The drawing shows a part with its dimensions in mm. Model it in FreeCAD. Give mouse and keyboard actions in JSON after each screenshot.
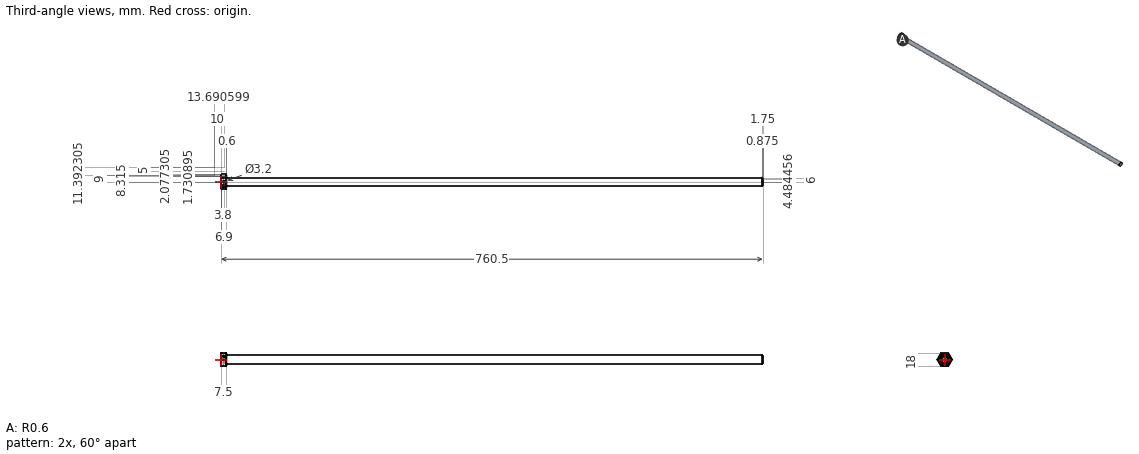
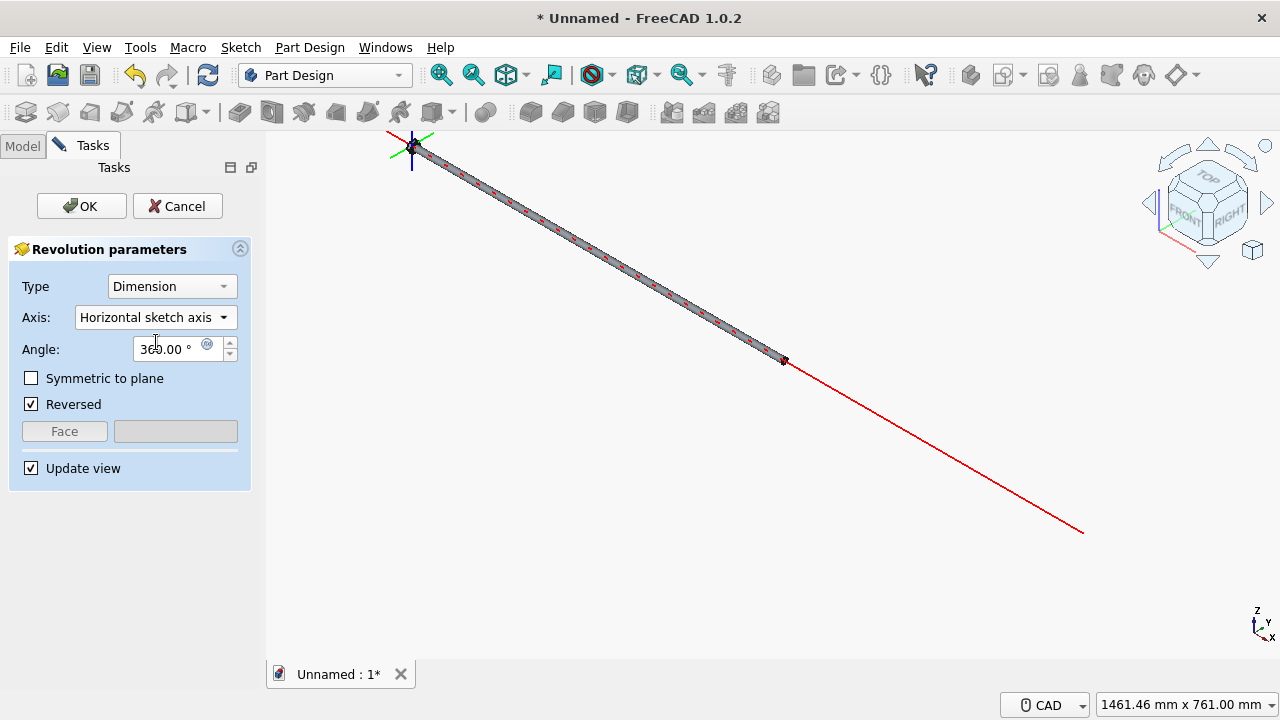
{"action": "left_click", "coordinate": [82, 206]}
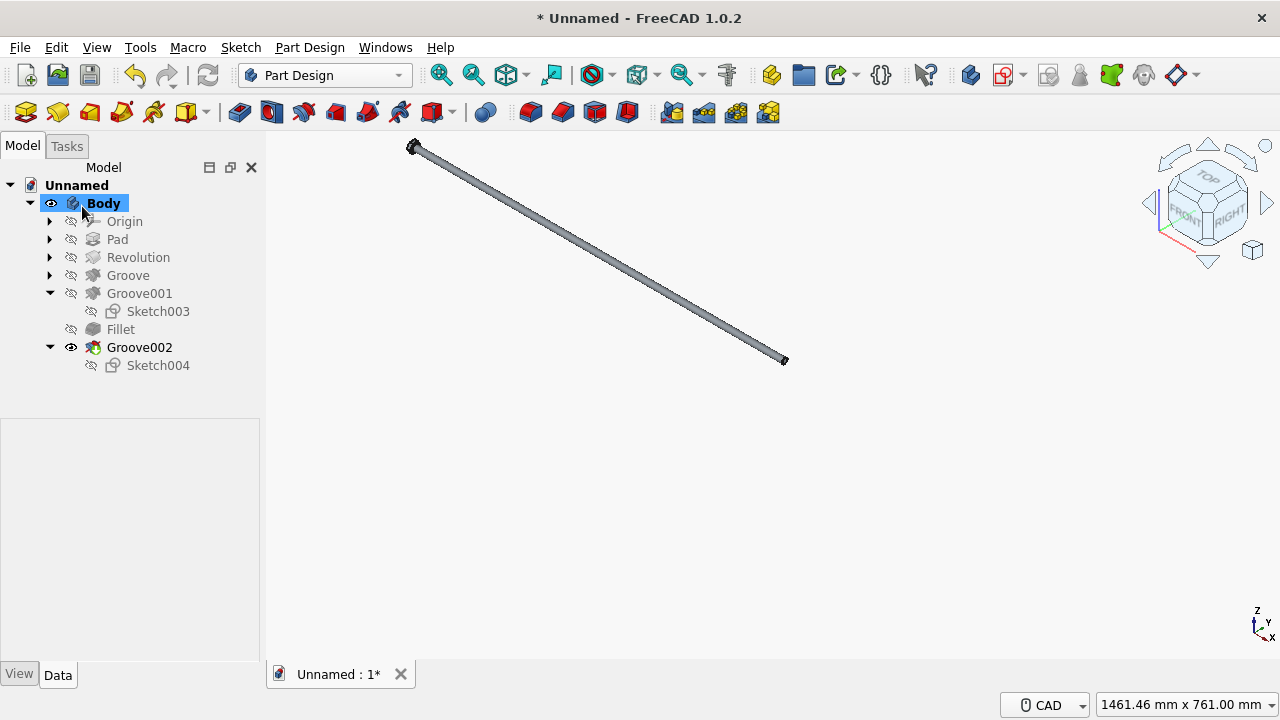
{"action": "key", "text": "v f"}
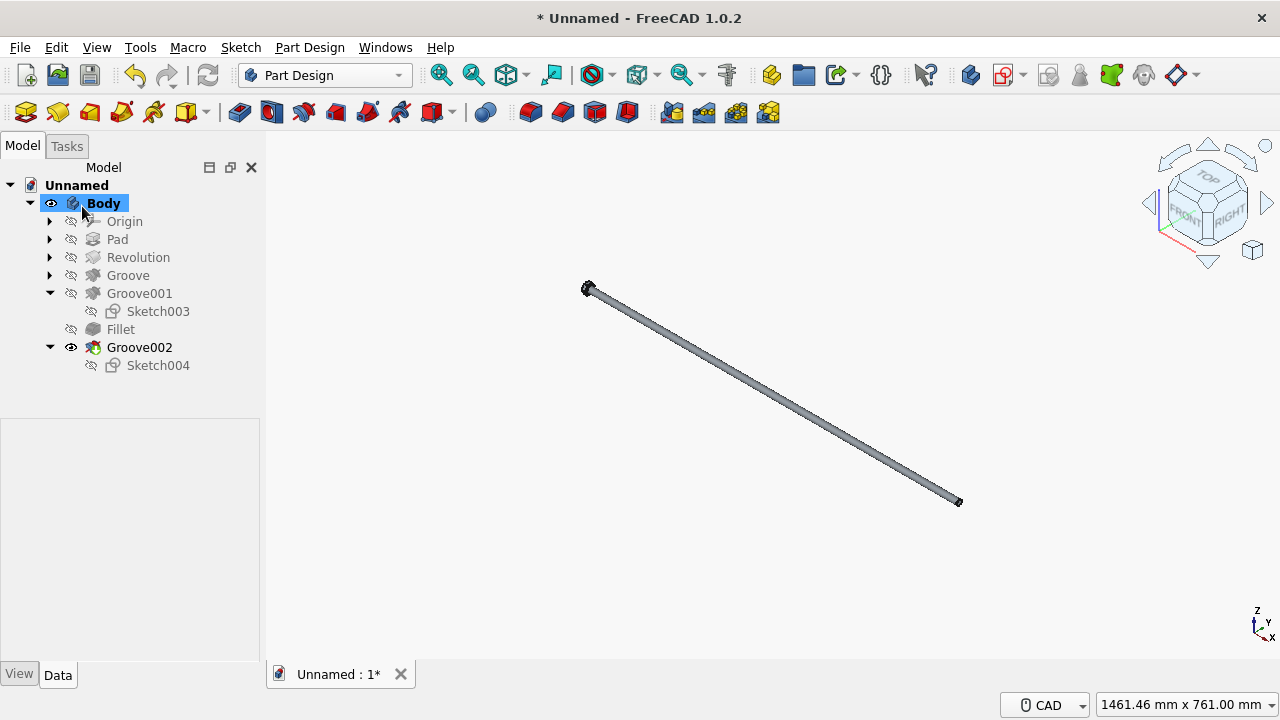
{"action": "left_click", "coordinate": [1004, 76]}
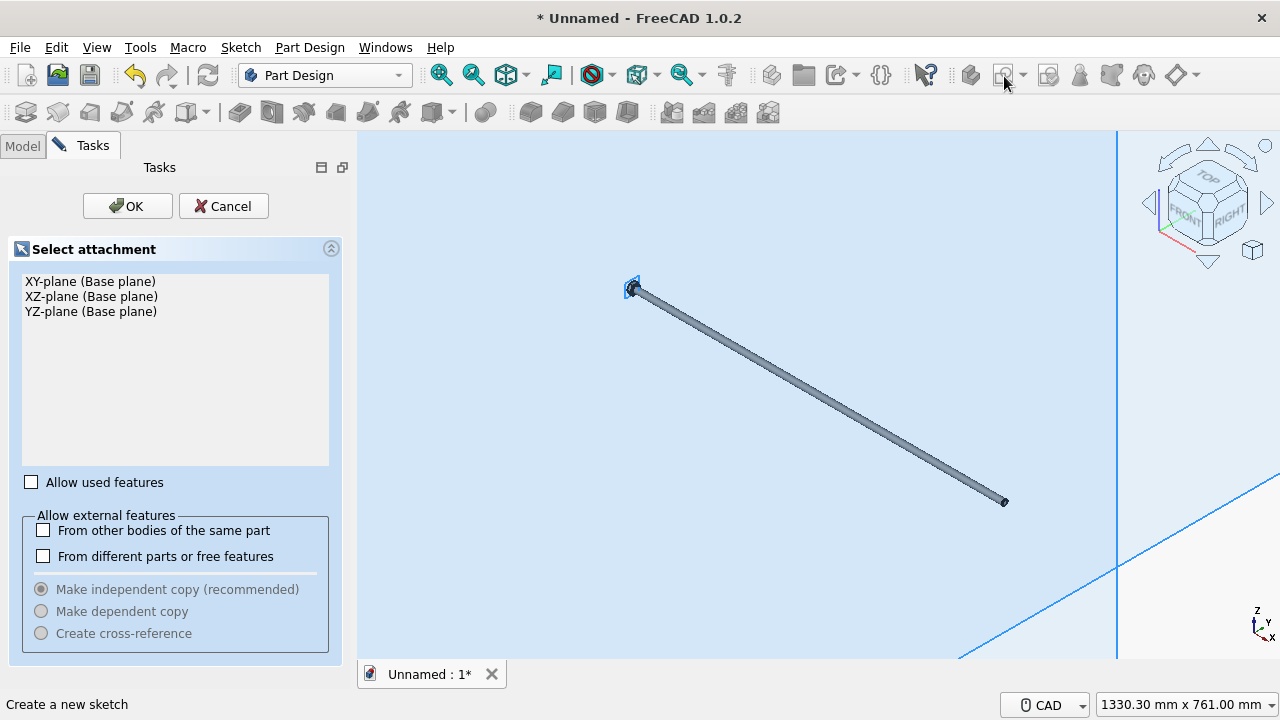
{"action": "left_click", "coordinate": [82, 282]}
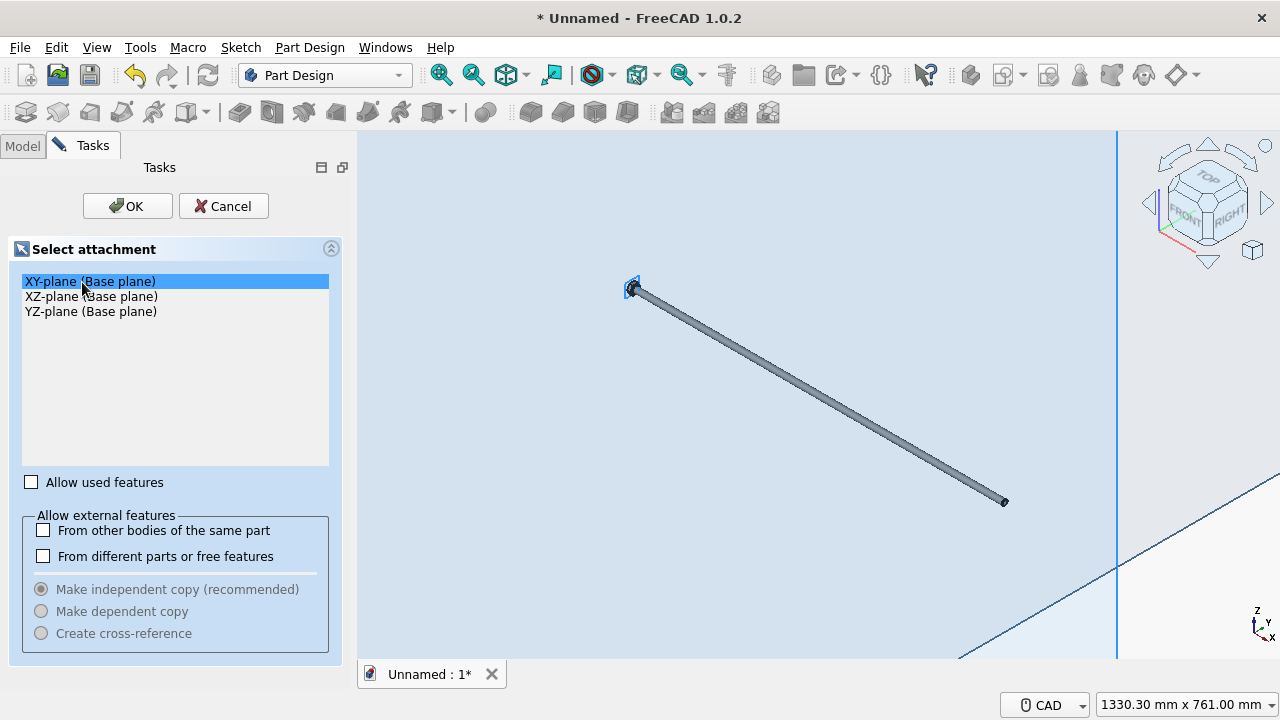
{"action": "left_click", "coordinate": [128, 206]}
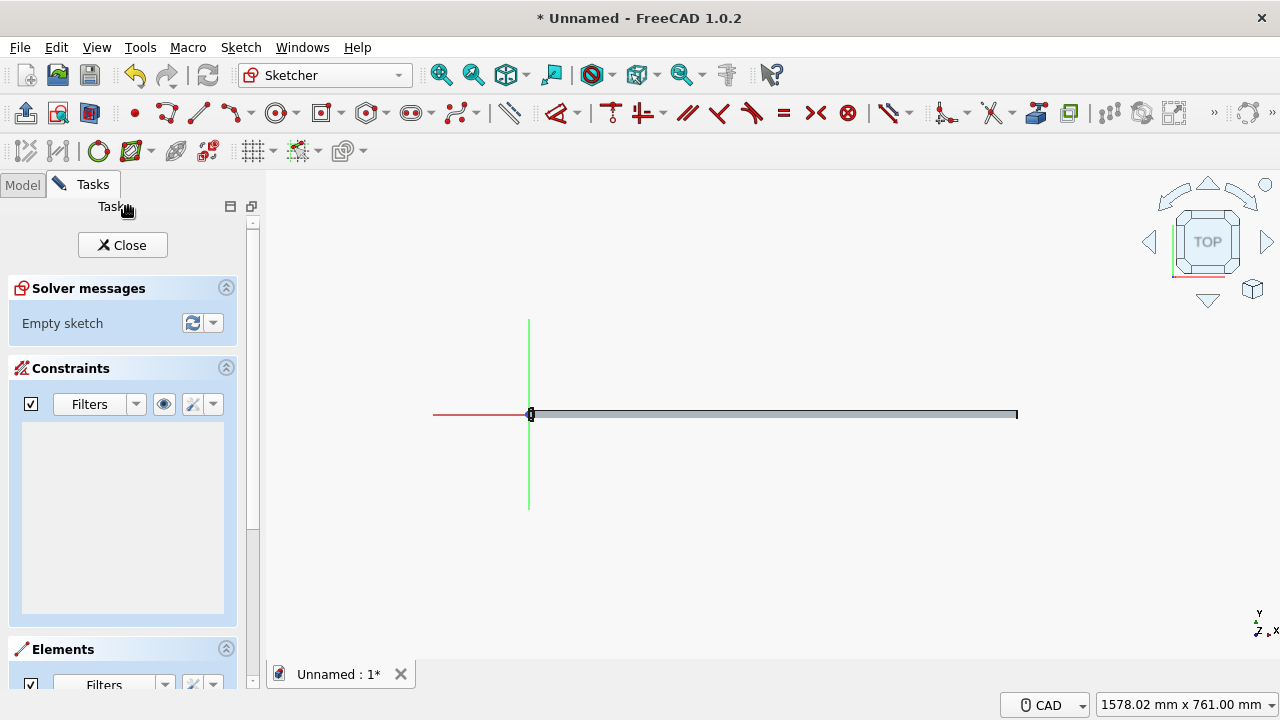
{"action": "key", "text": "q s"}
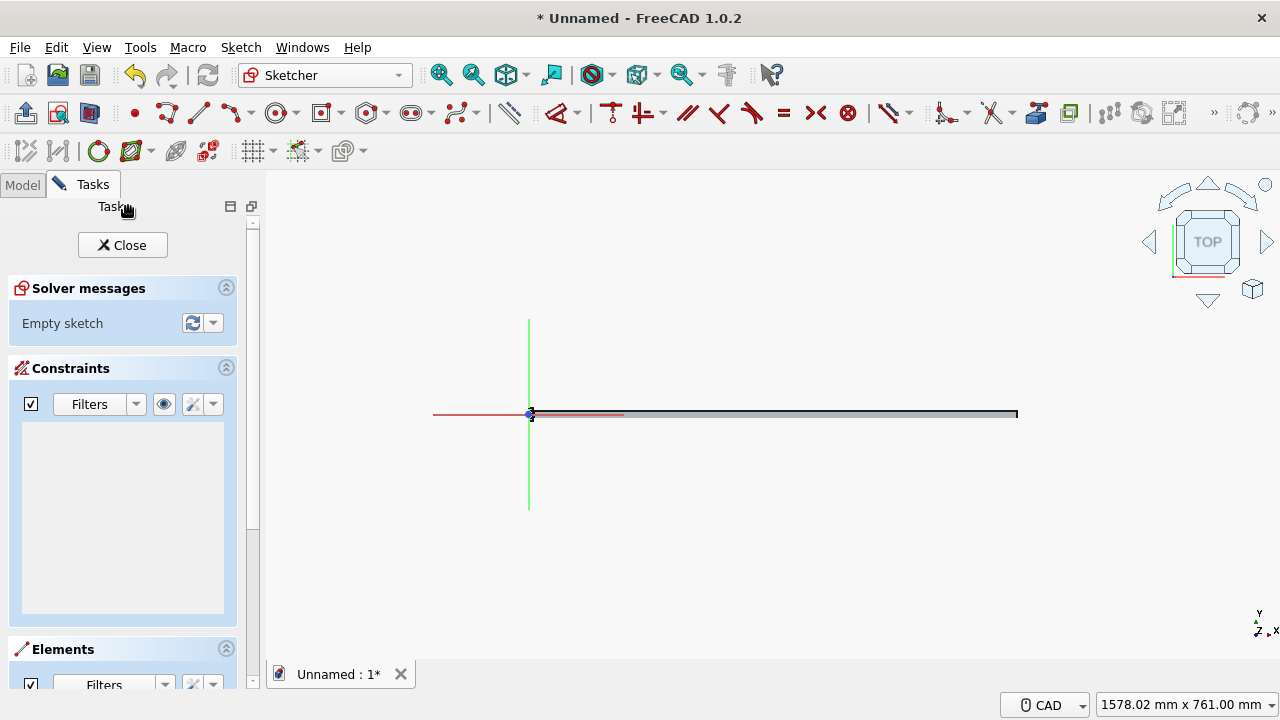
{"action": "scroll", "coordinate": [521, 414], "scroll_direction": "up", "scroll_amount": 15}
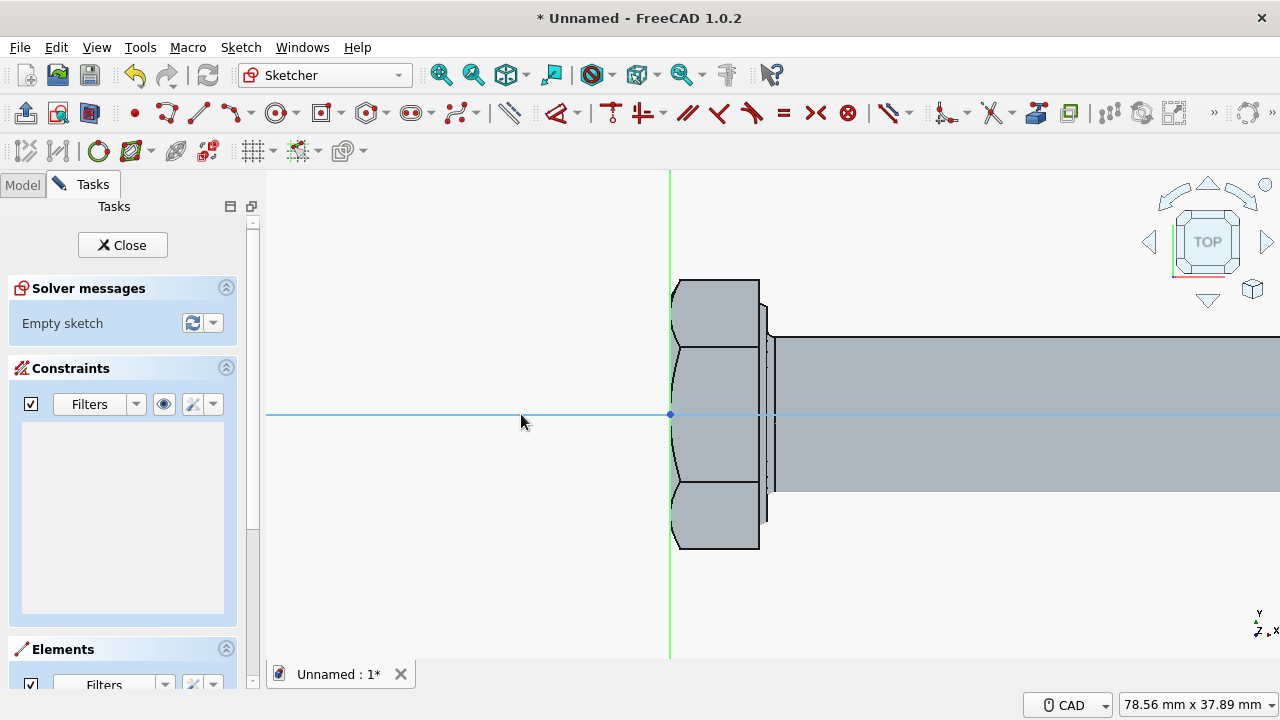
{"action": "scroll", "coordinate": [705, 414], "scroll_direction": "up", "scroll_amount": 10}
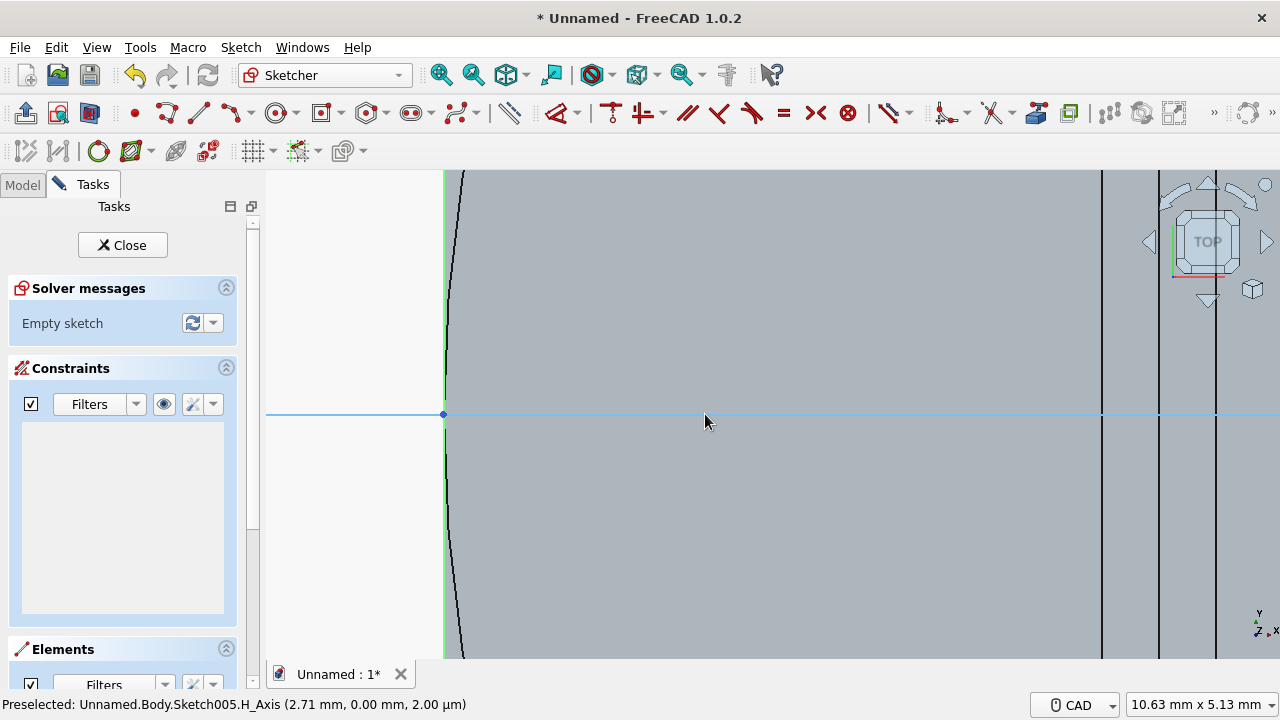
{"action": "key", "text": "g c"}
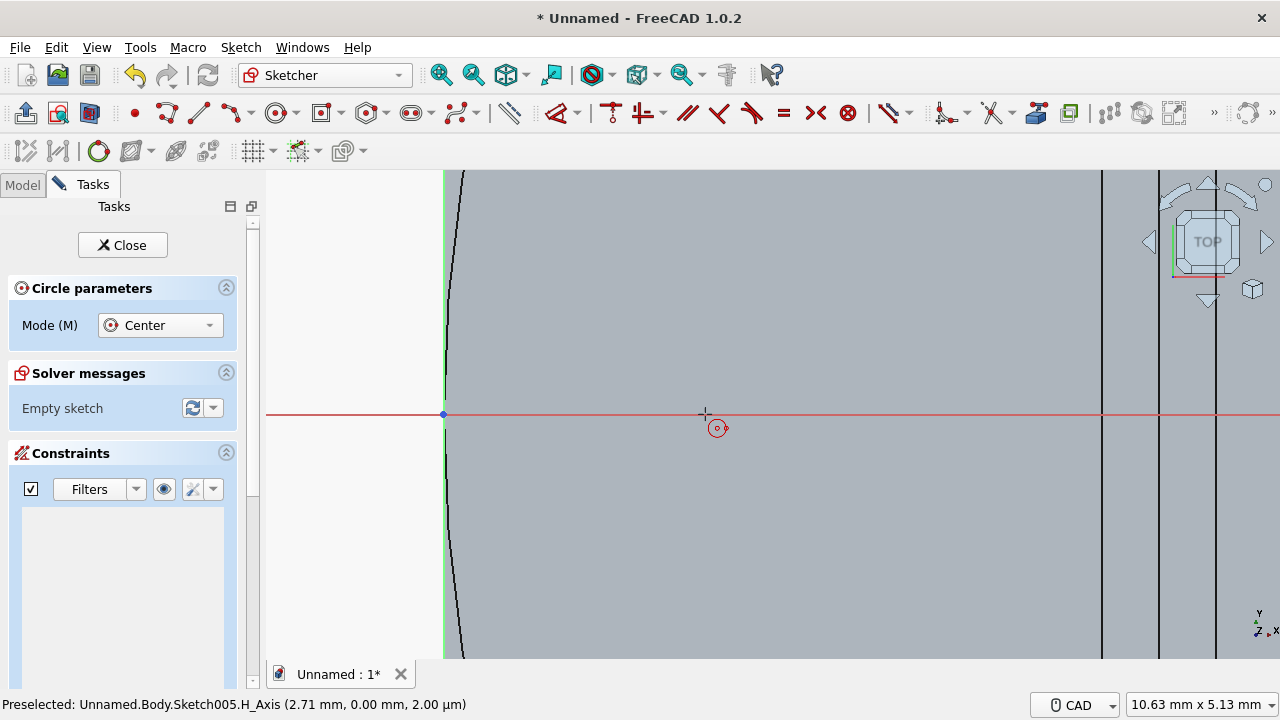
{"action": "left_click", "coordinate": [806, 414]}
{"action": "mouse_move", "coordinate": [914, 307]}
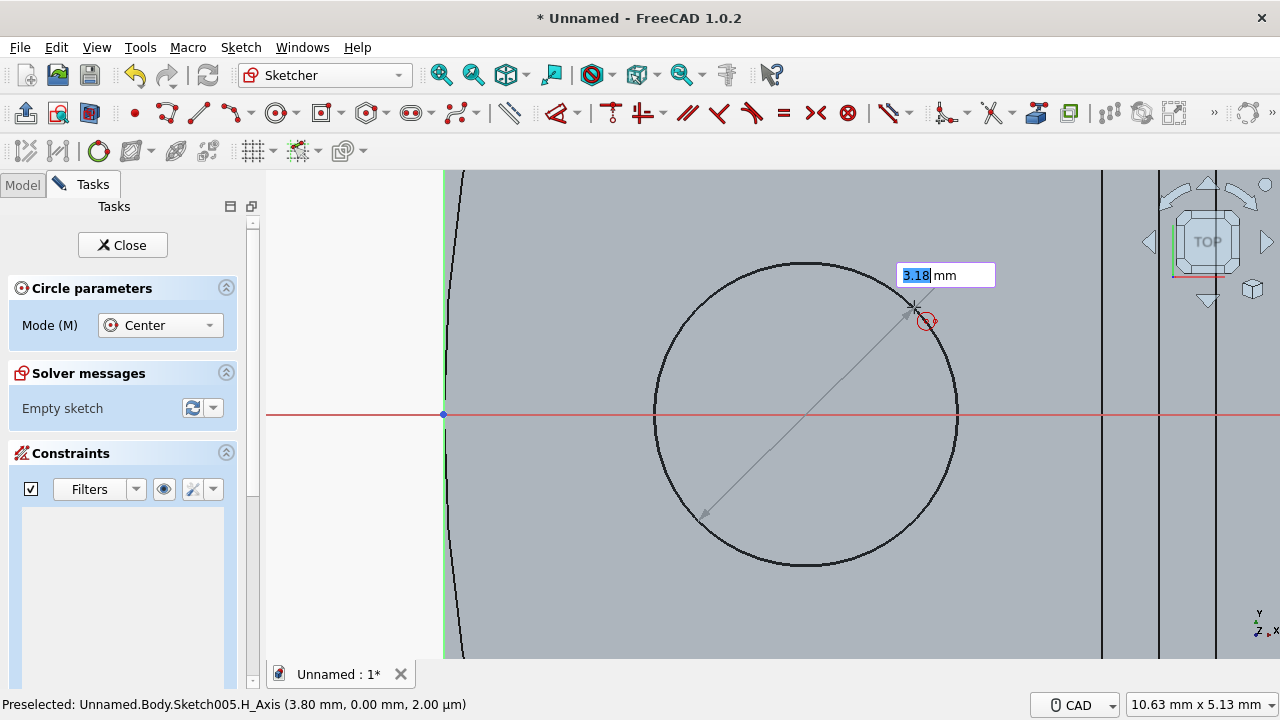
{"action": "type", "text": "3.2"}
{"action": "key", "text": "Return"}
{"action": "key", "text": "Escape"}